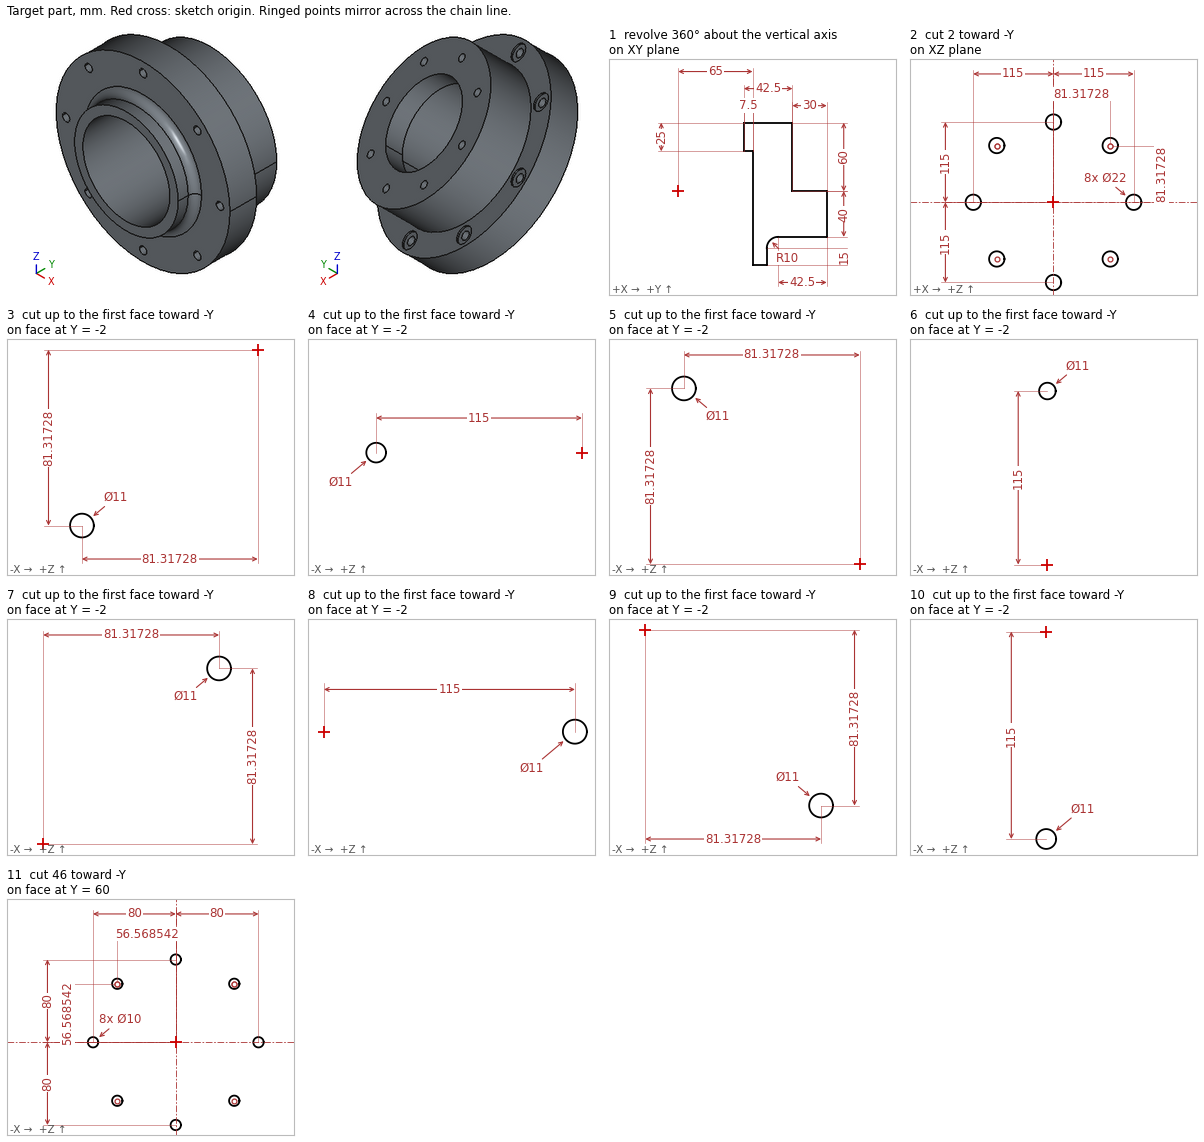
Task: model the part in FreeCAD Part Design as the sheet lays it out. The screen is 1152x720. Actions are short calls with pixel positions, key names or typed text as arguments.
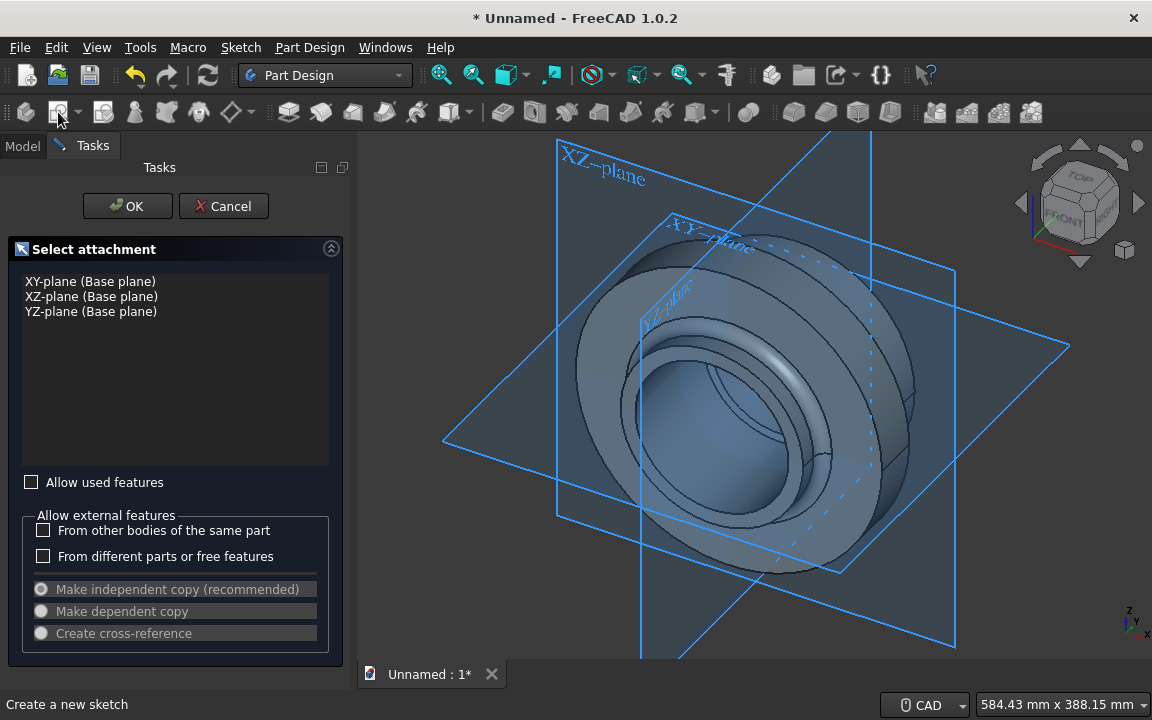
click(82, 296)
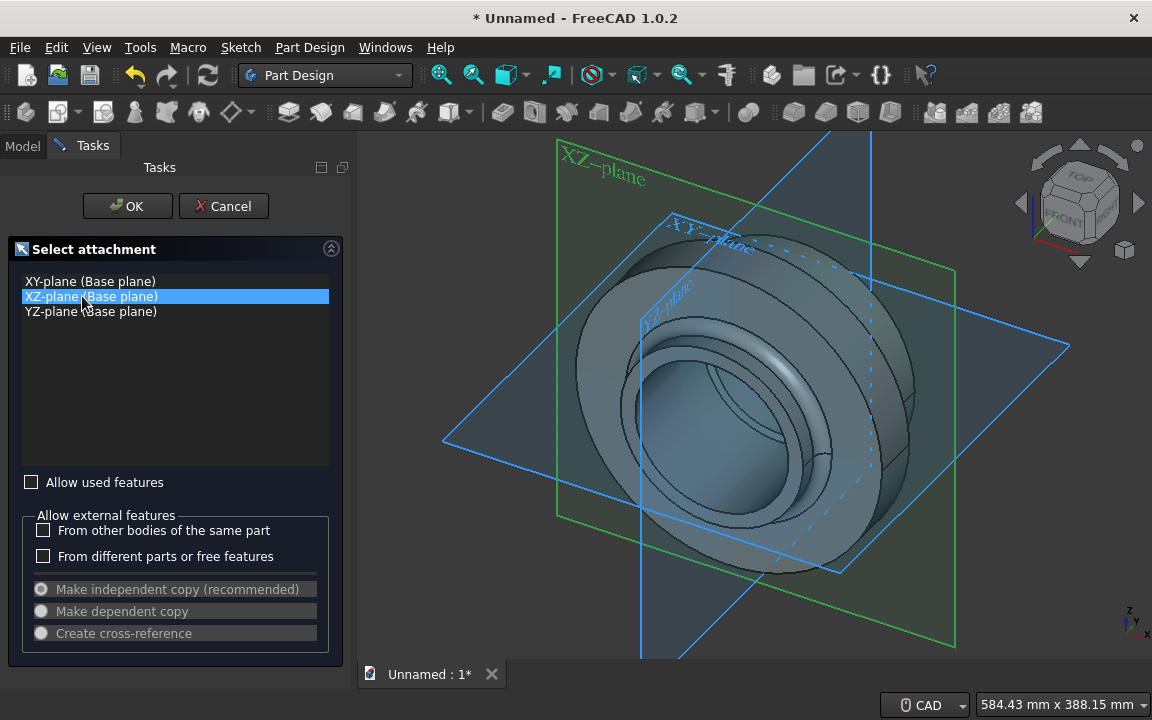
click(128, 206)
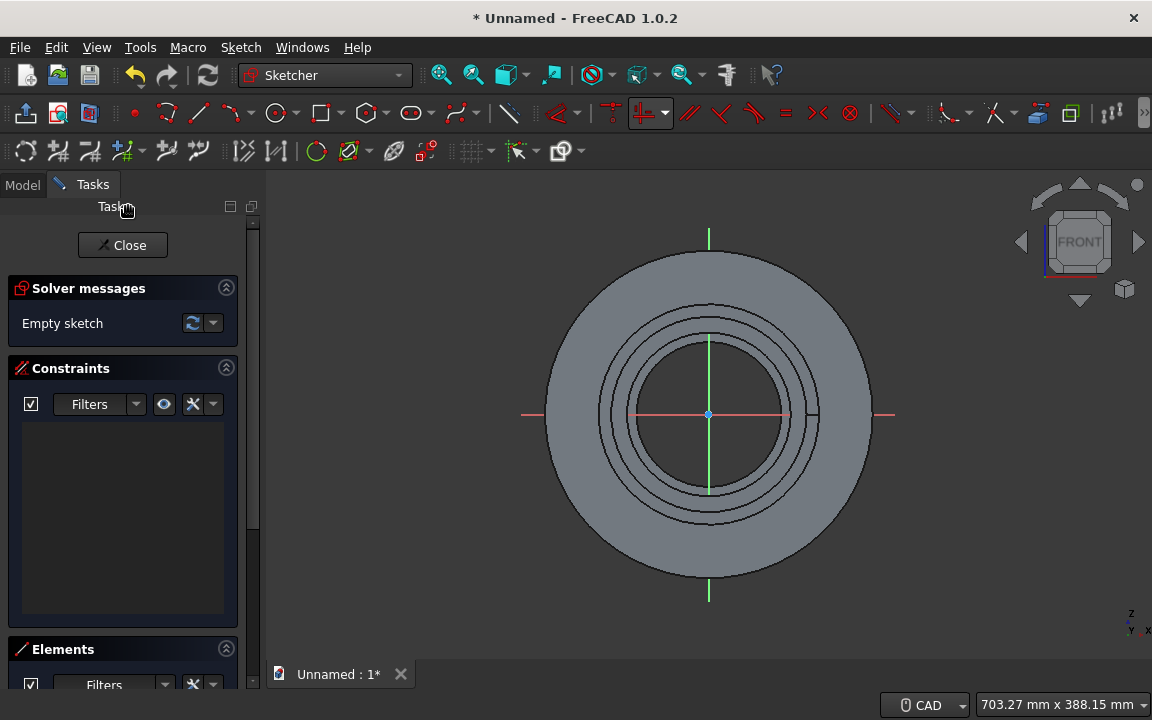
key(q)
key(s)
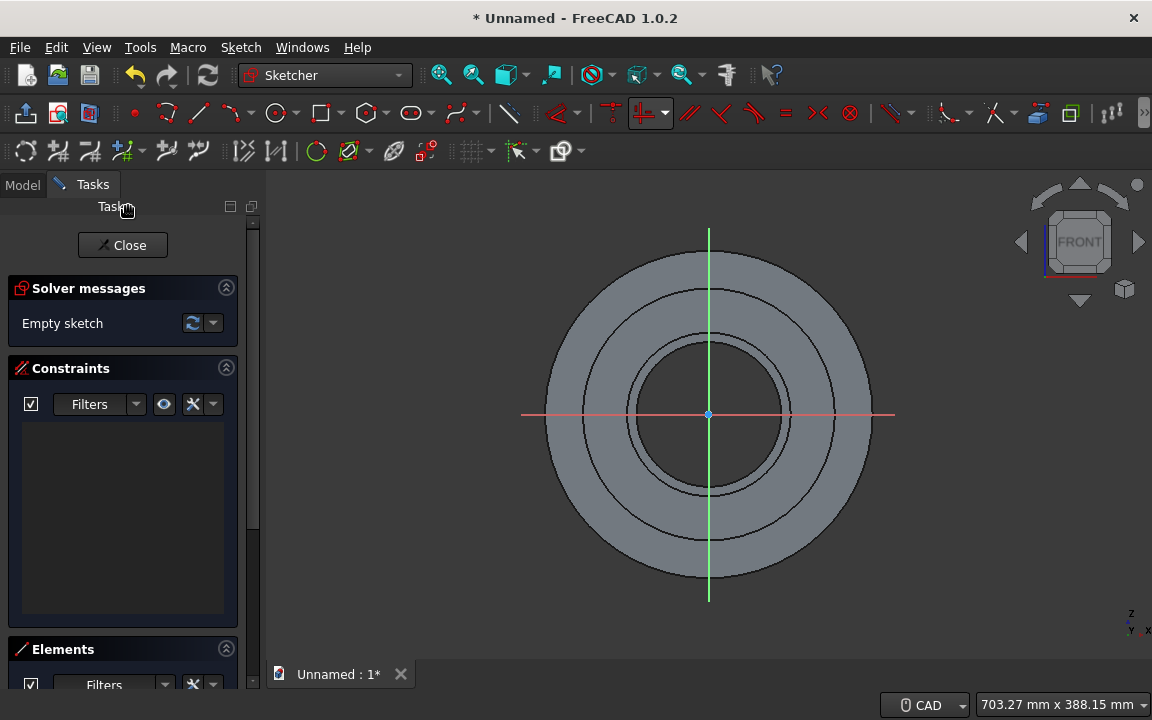
click(276, 114)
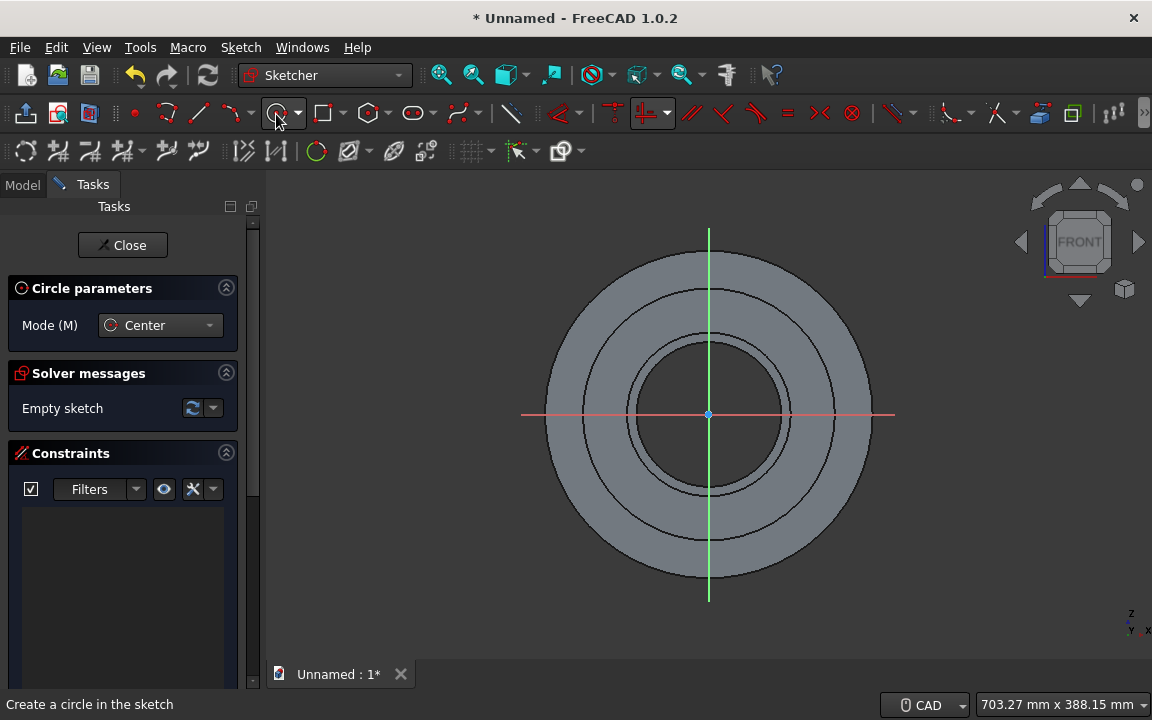
scroll(854, 414, up, 3)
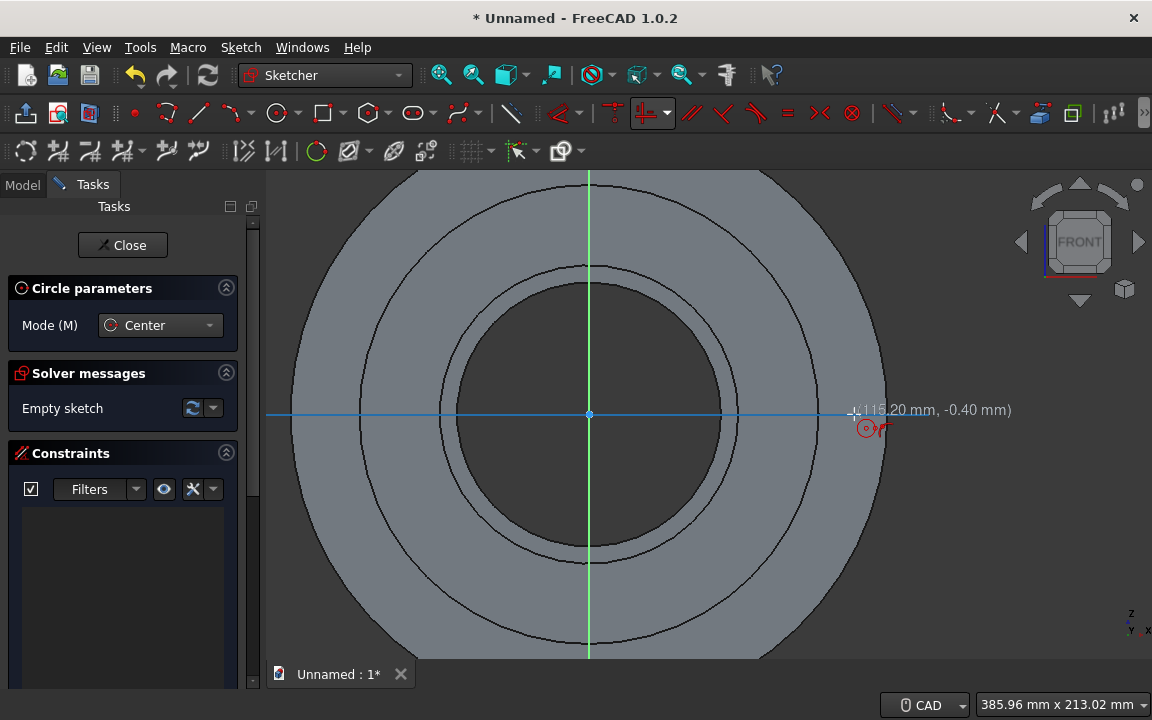
click(853, 414)
move(871, 397)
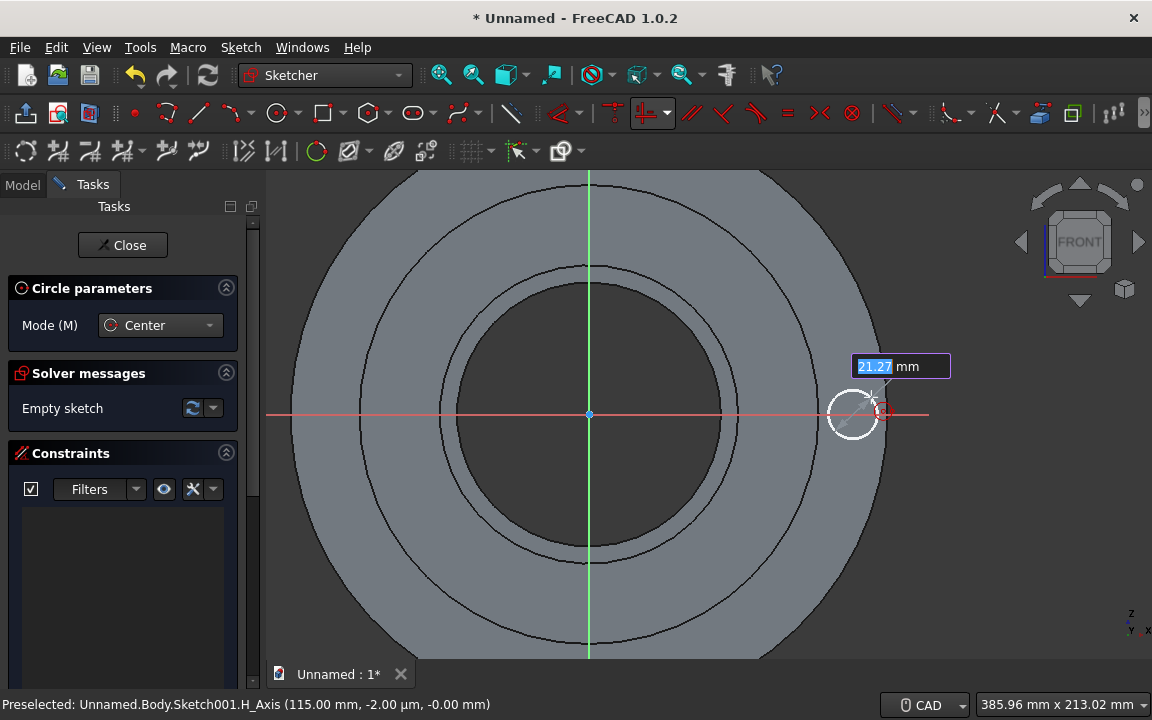
text(22)
key(Return)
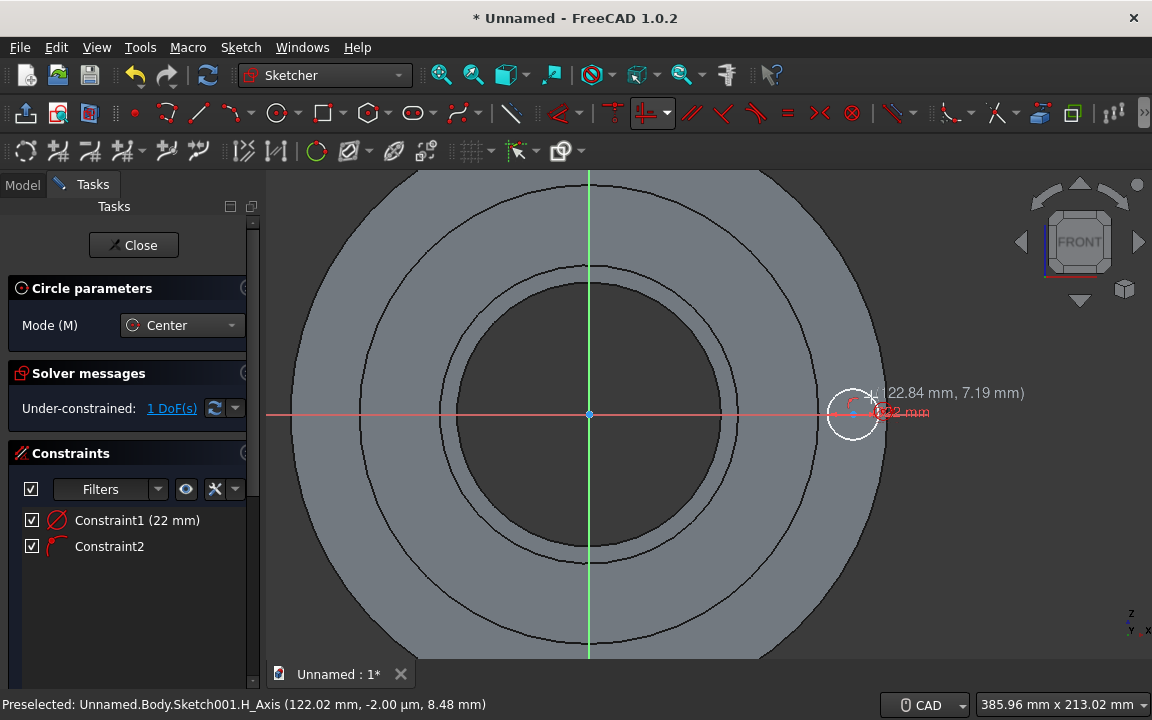
click(776, 228)
move(794, 210)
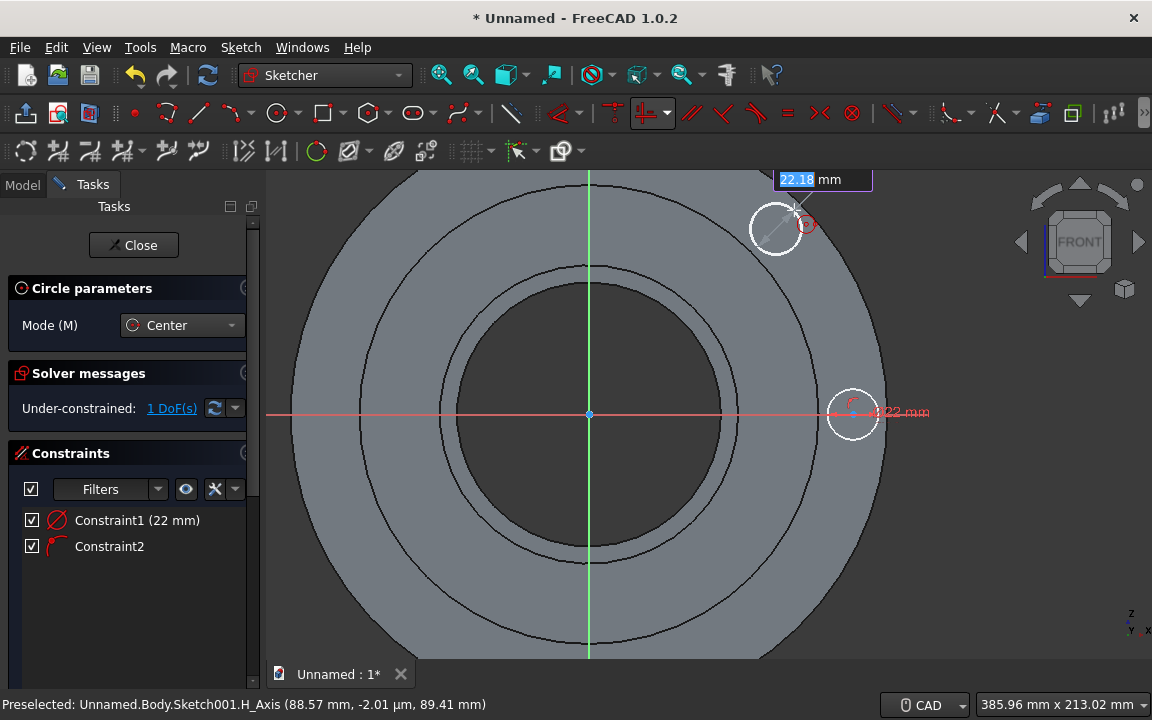
text(22)
key(Return)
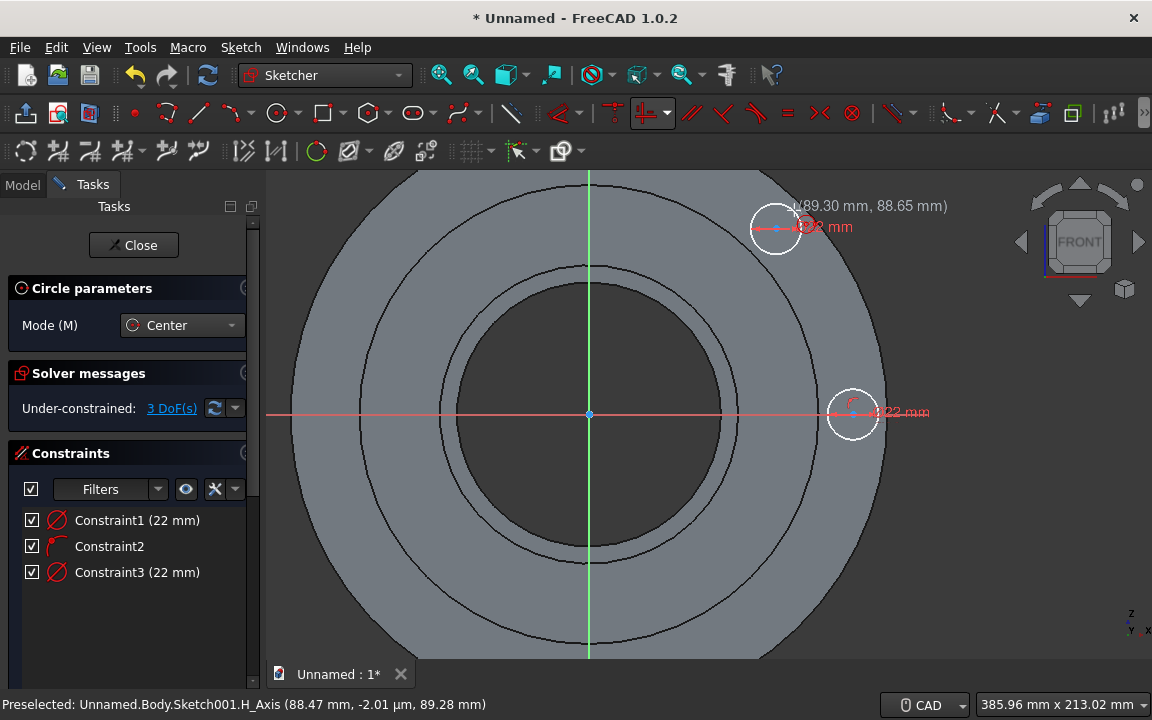
scroll(703, 414, down, 3)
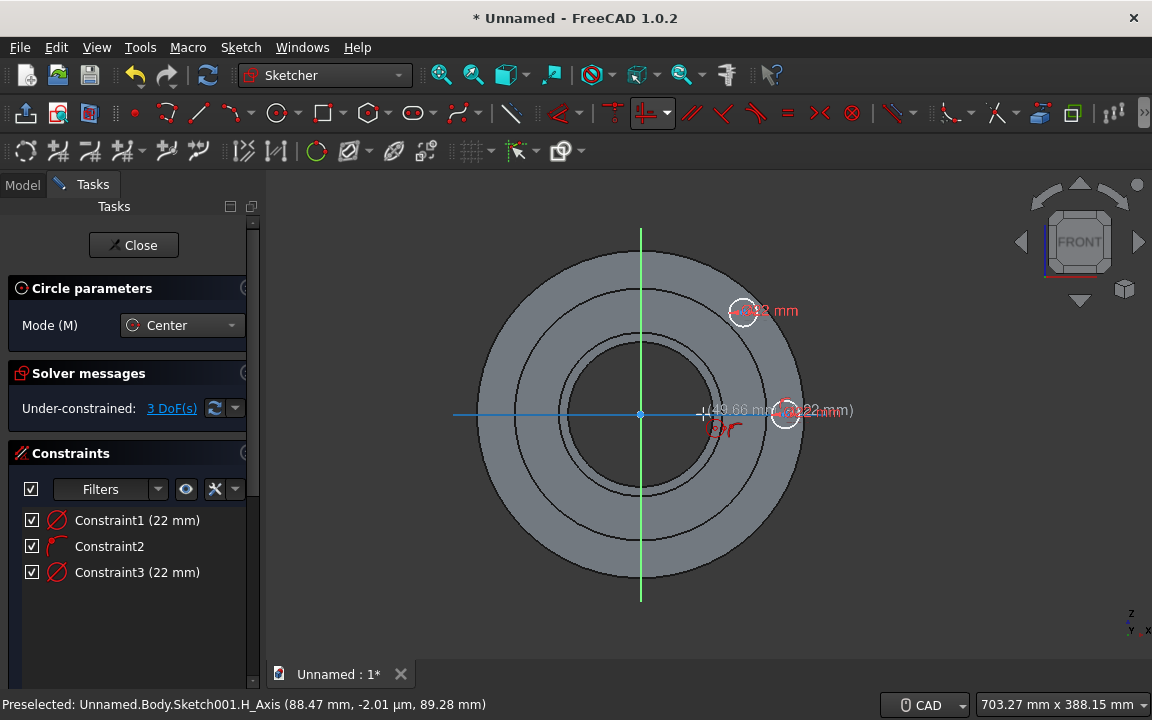
scroll(641, 270, up, 3)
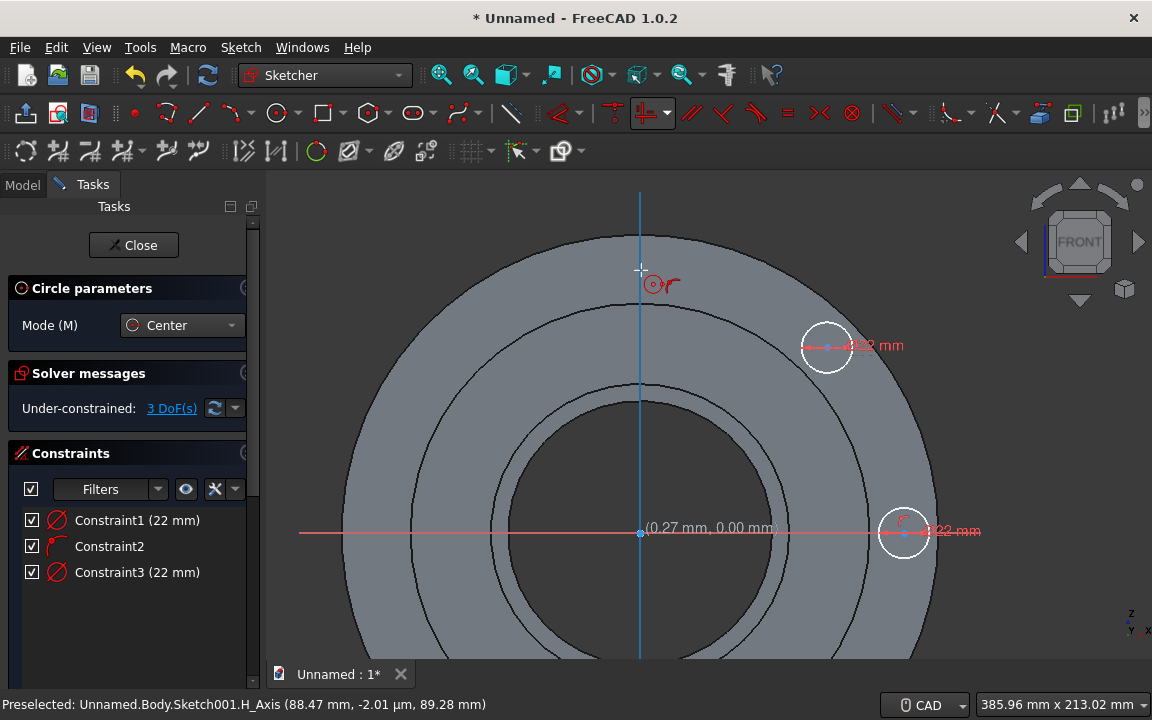
click(640, 269)
move(658, 251)